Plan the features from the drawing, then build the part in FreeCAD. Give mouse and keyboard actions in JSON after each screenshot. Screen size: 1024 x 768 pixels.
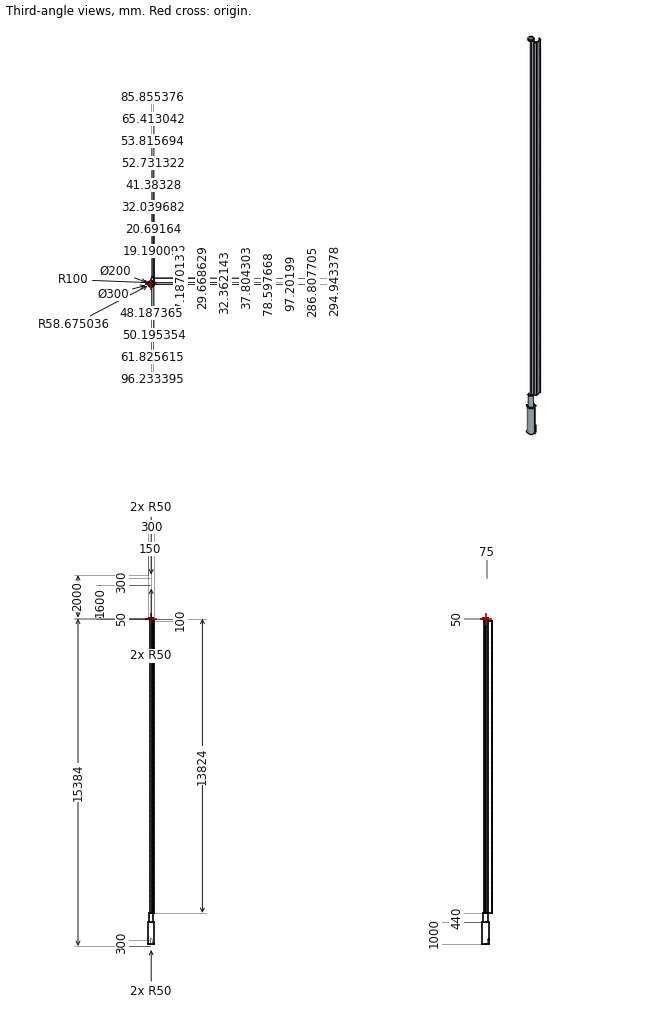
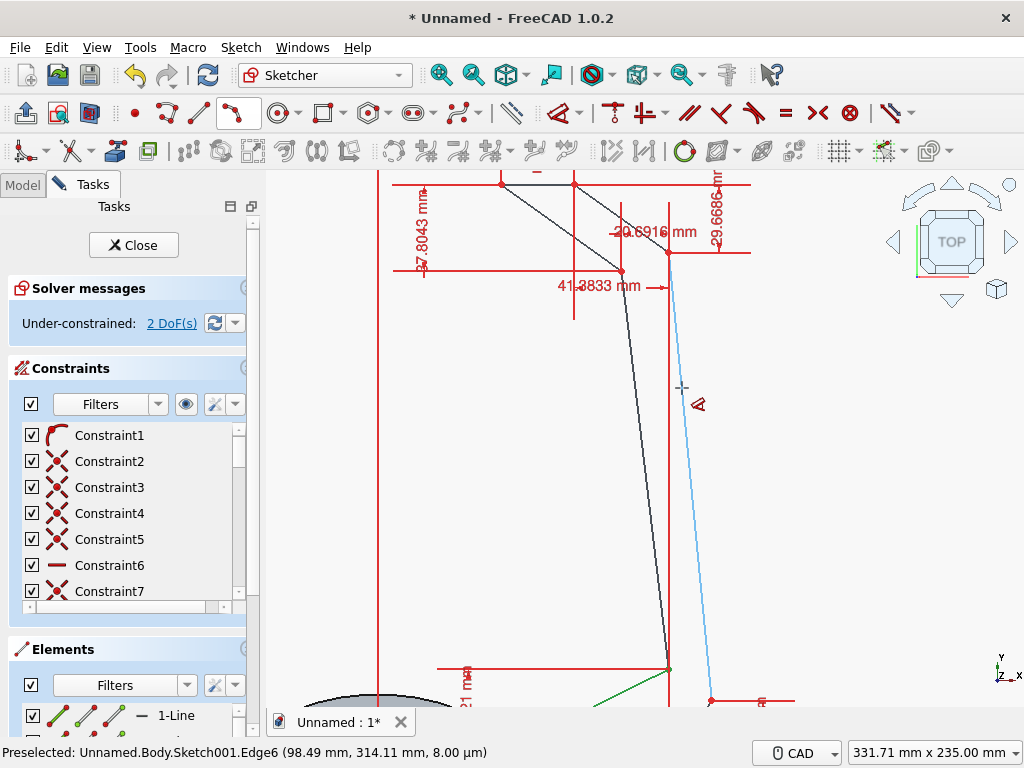
{"action": "left_click", "coordinate": [682, 387]}
{"action": "left_click", "coordinate": [690, 219]}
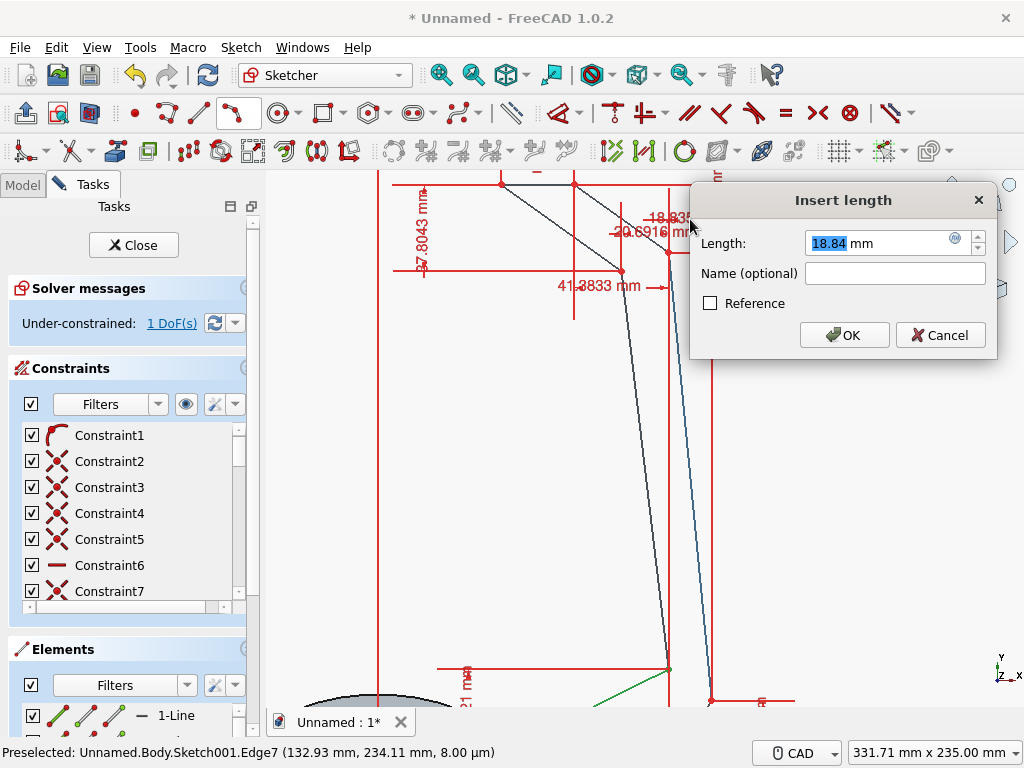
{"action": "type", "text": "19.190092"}
{"action": "key", "text": "Return"}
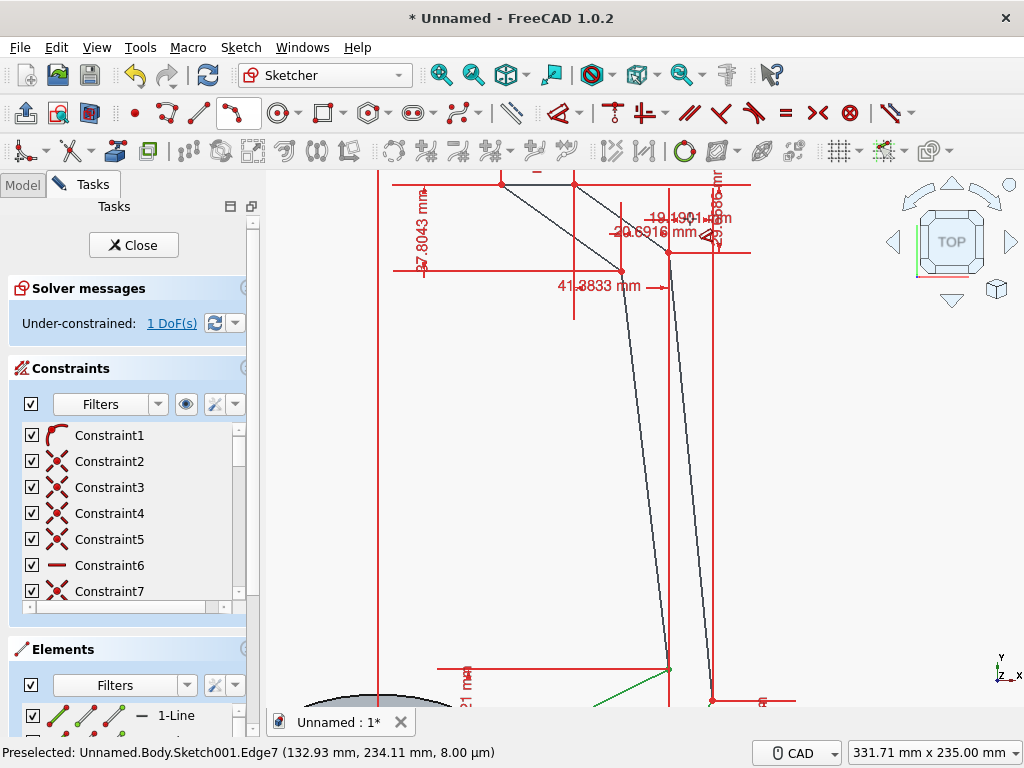
{"action": "left_click", "coordinate": [622, 271]}
{"action": "left_click", "coordinate": [656, 381]}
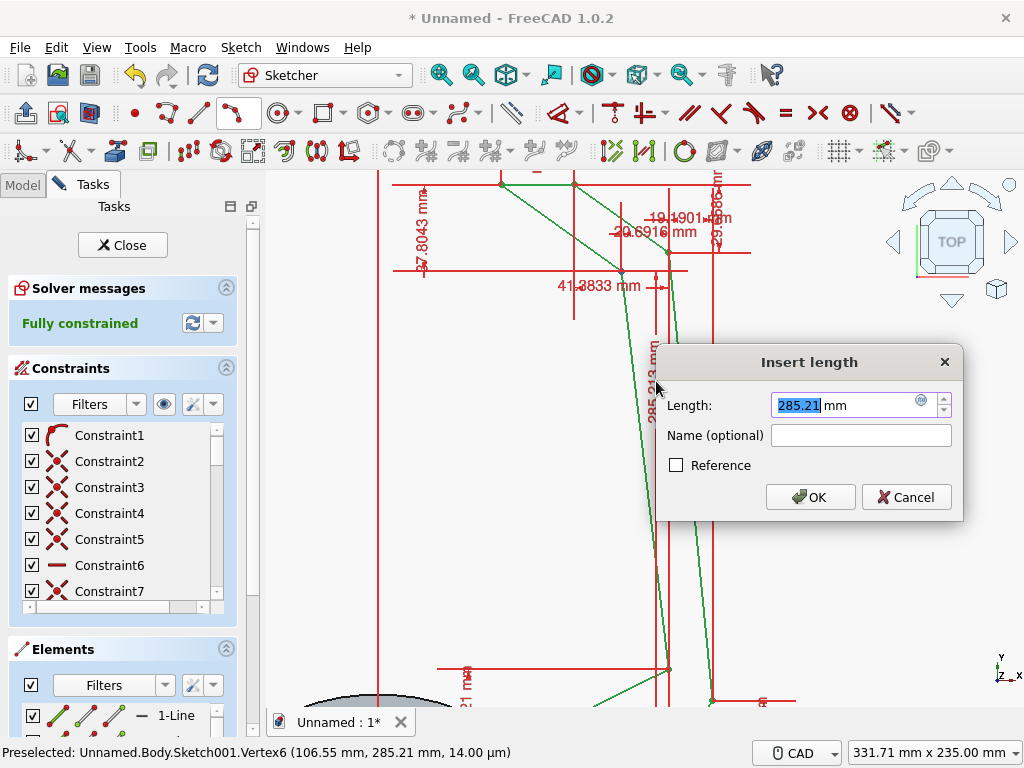
{"action": "type", "text": "286.807705"}
{"action": "key", "text": "Return"}
{"action": "key", "text": "Escape"}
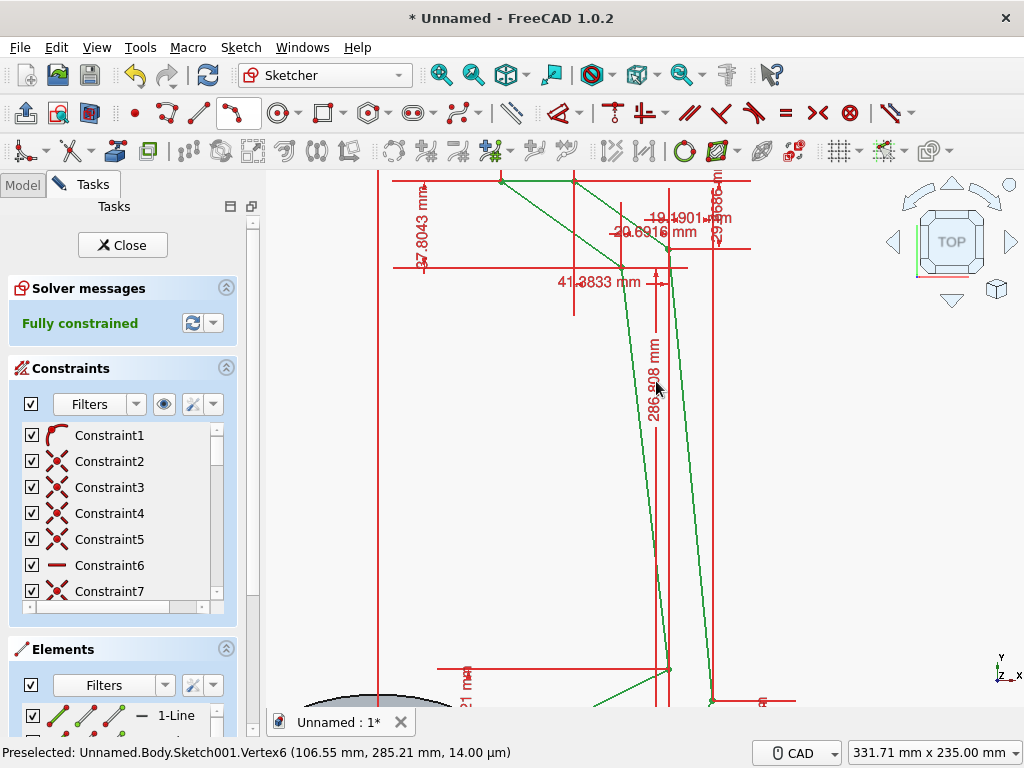
{"action": "left_click", "coordinate": [123, 245]}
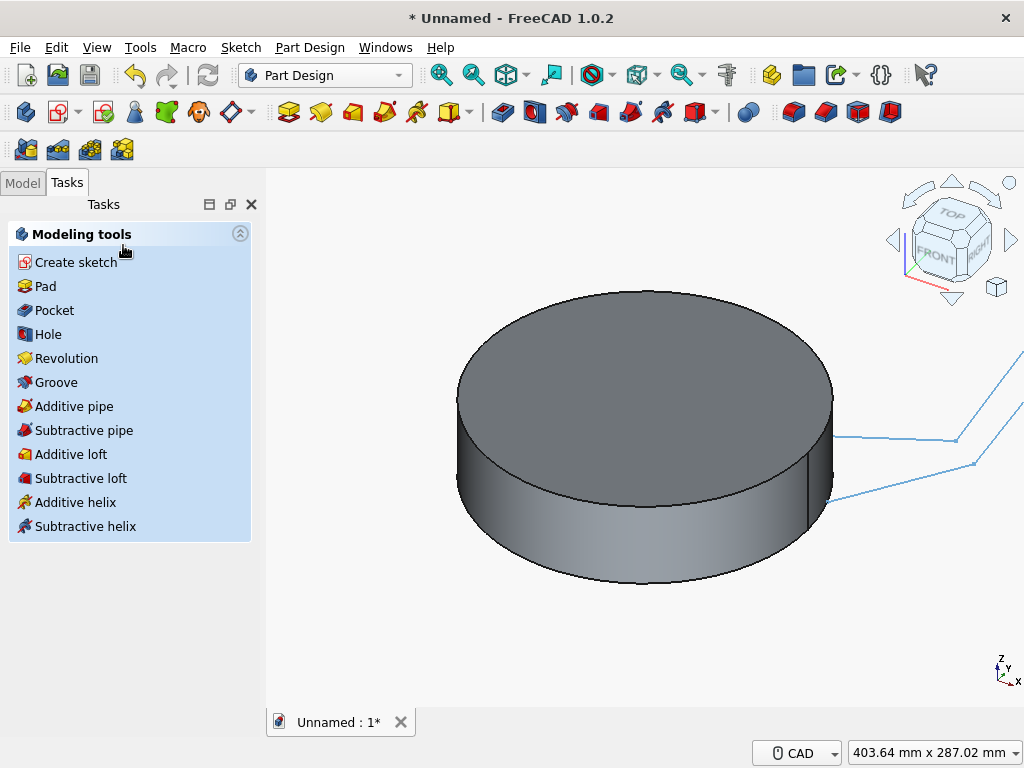
{"action": "left_click", "coordinate": [290, 112]}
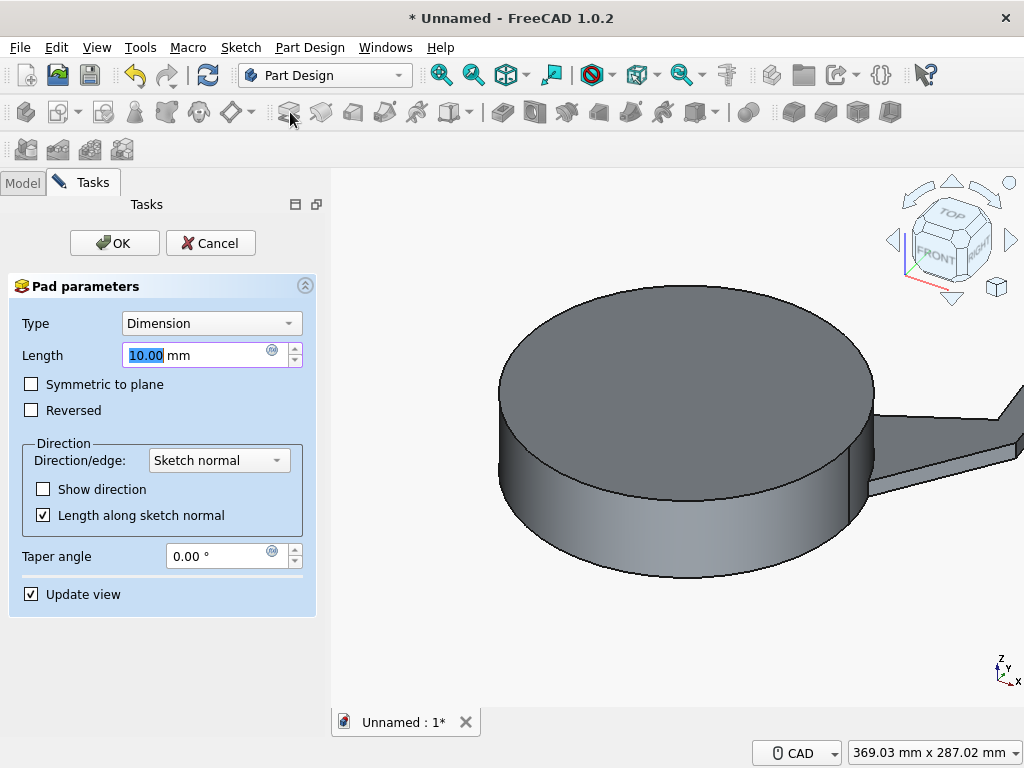
{"action": "type", "text": "13824"}
{"action": "key", "text": "Tab"}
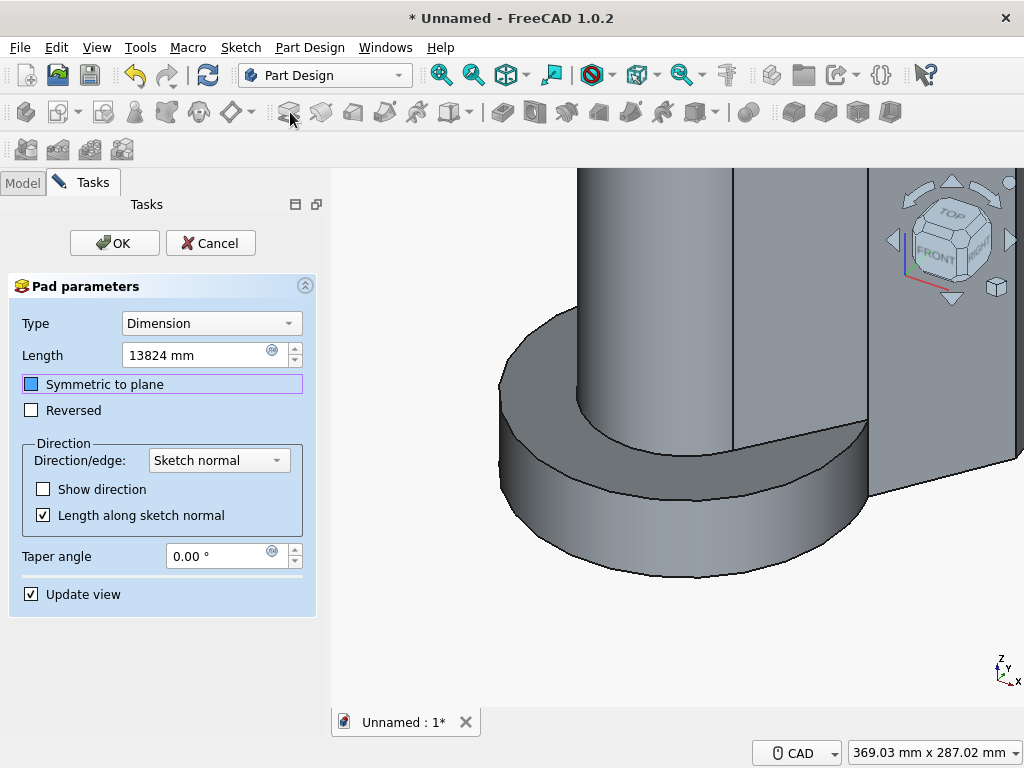
{"action": "left_click", "coordinate": [30, 410]}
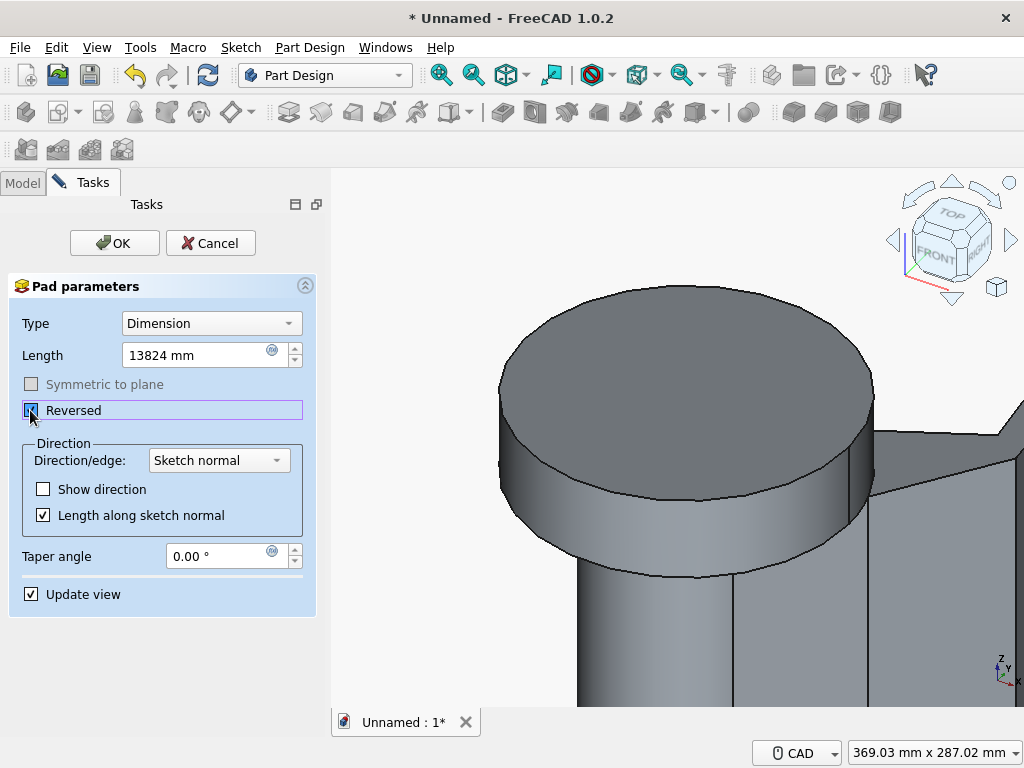
{"action": "left_click", "coordinate": [115, 243]}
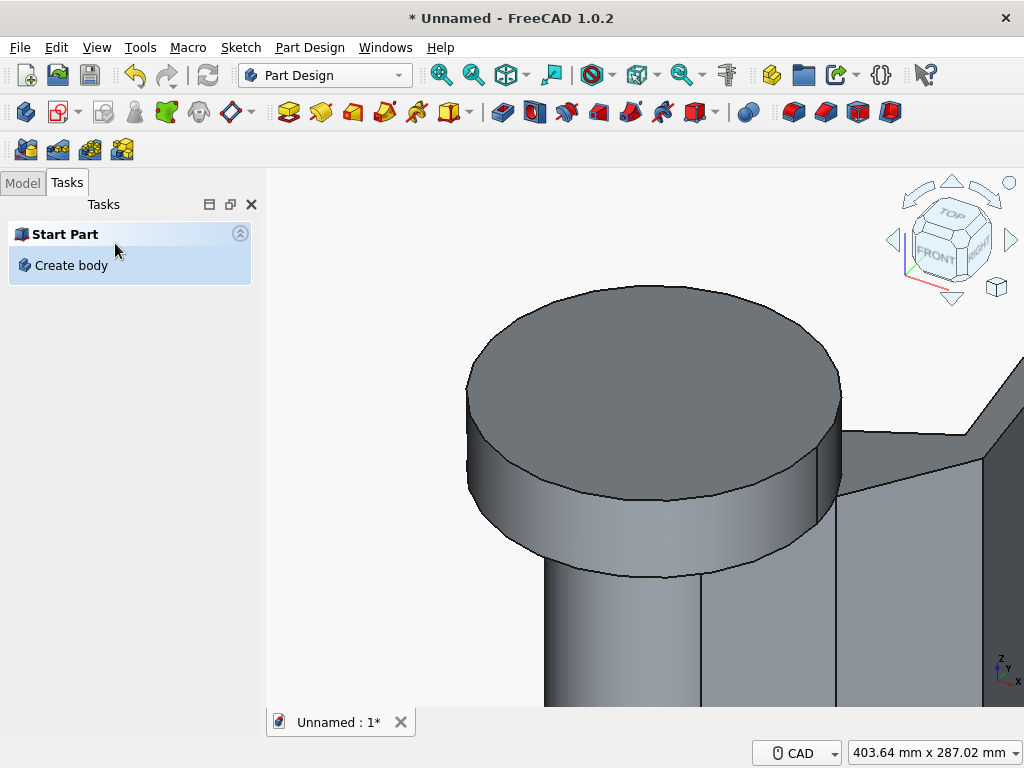
{"action": "left_click", "coordinate": [442, 76]}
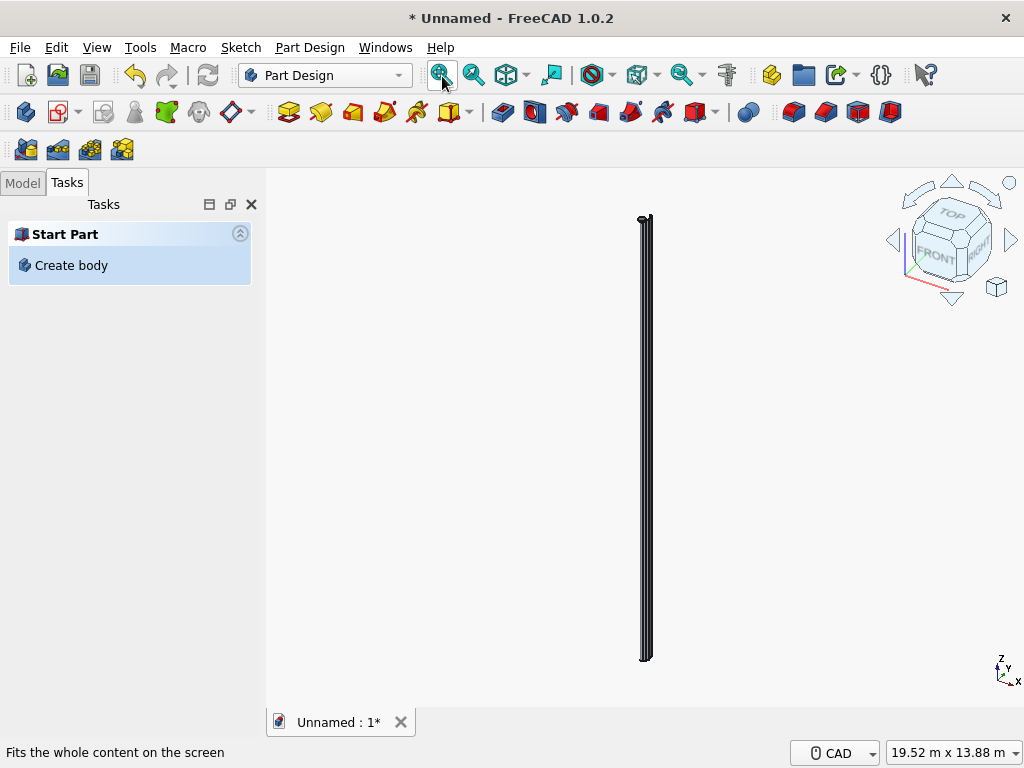
{"action": "left_click", "coordinate": [23, 182]}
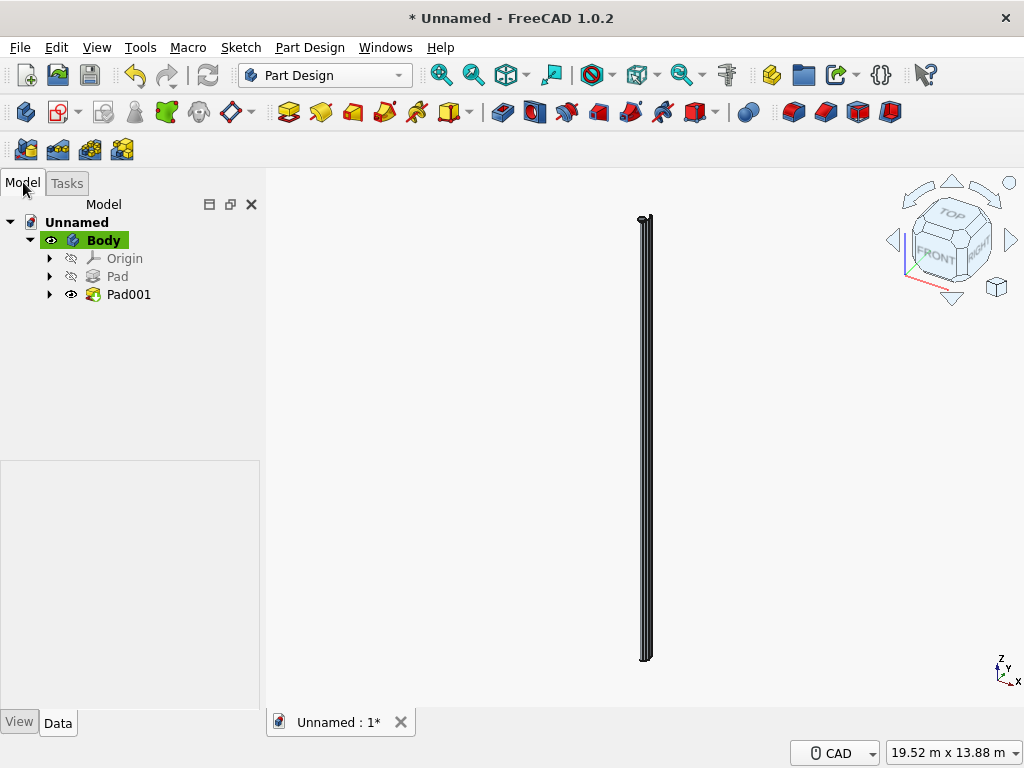
{"action": "left_click", "coordinate": [50, 258]}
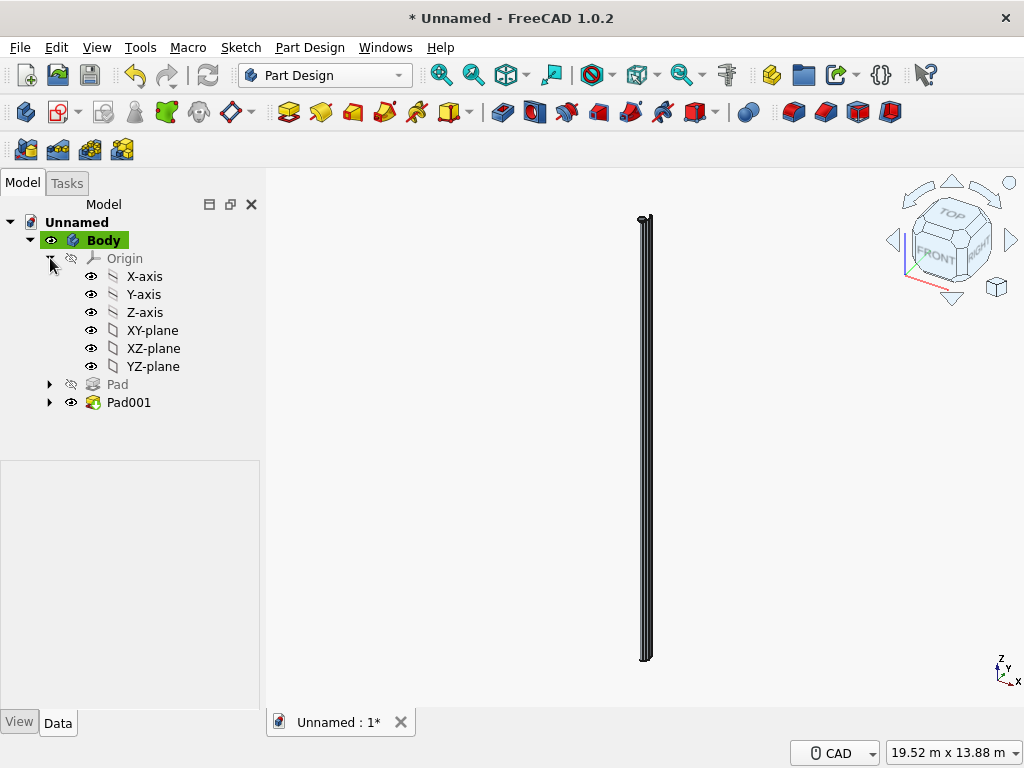
{"action": "left_click", "coordinate": [136, 330]}